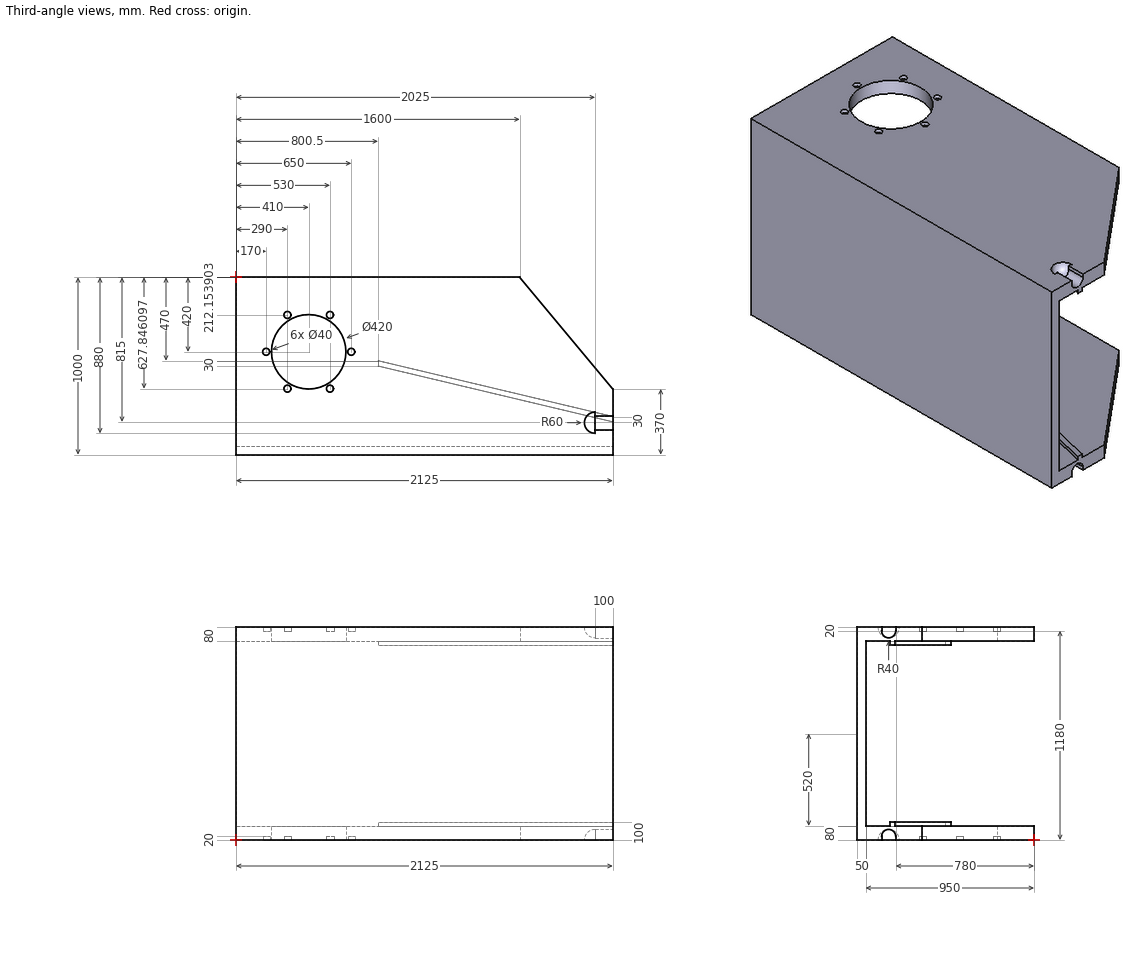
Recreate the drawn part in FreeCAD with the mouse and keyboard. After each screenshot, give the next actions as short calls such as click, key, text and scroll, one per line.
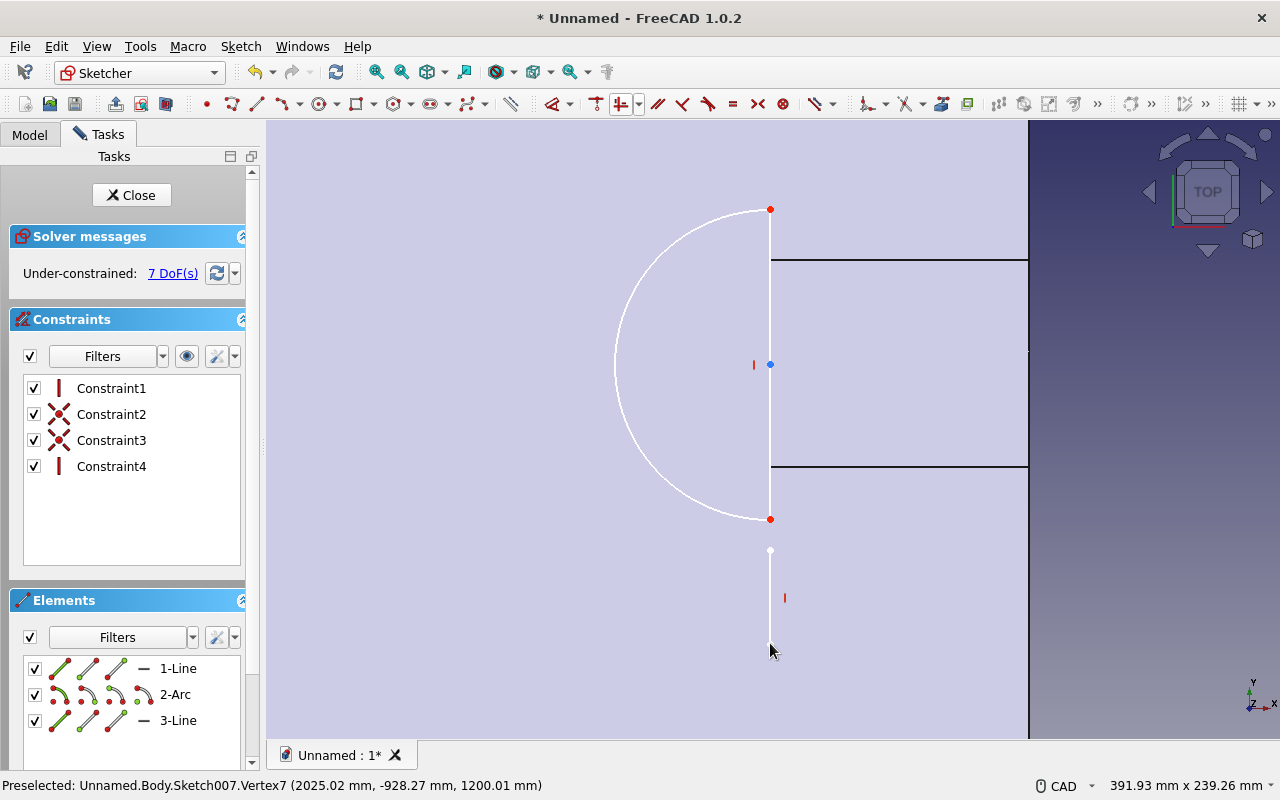
click(770, 579)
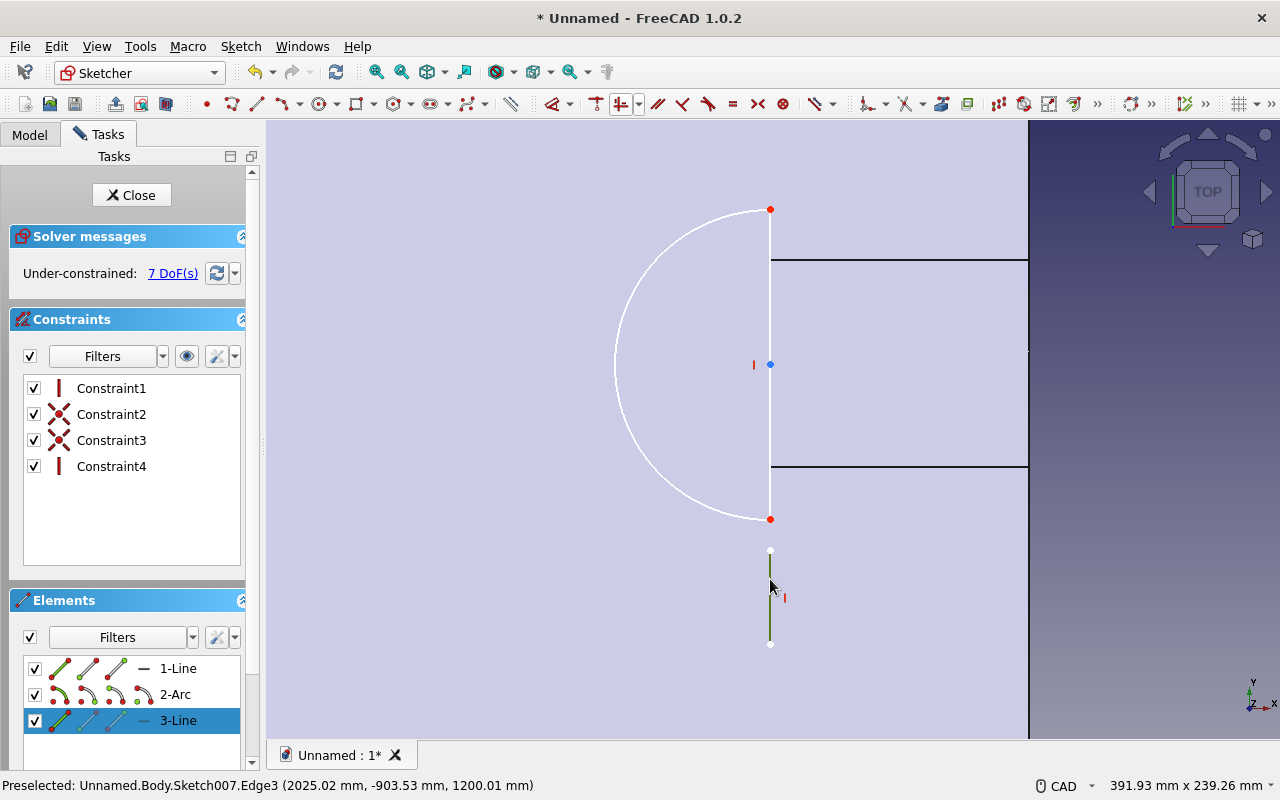
key(g)
key(n)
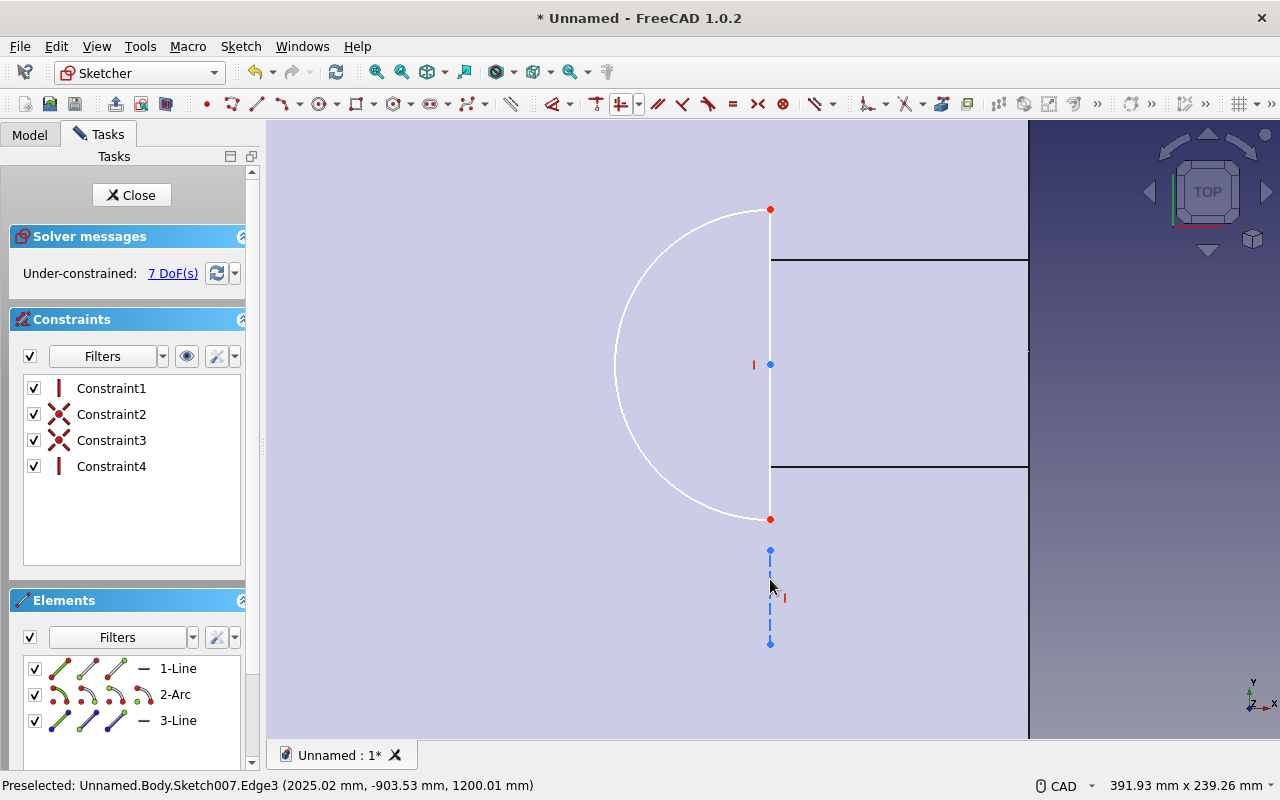
key(d)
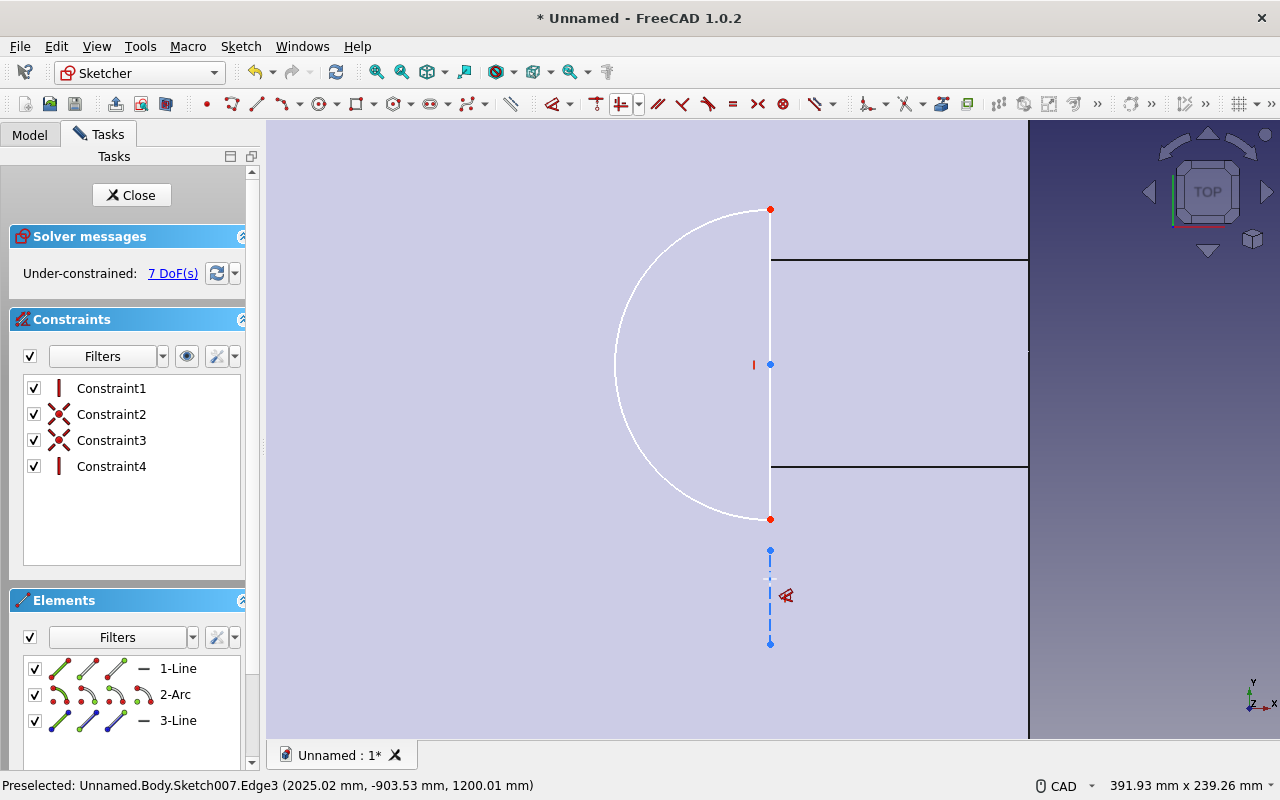
click(645, 274)
click(619, 255)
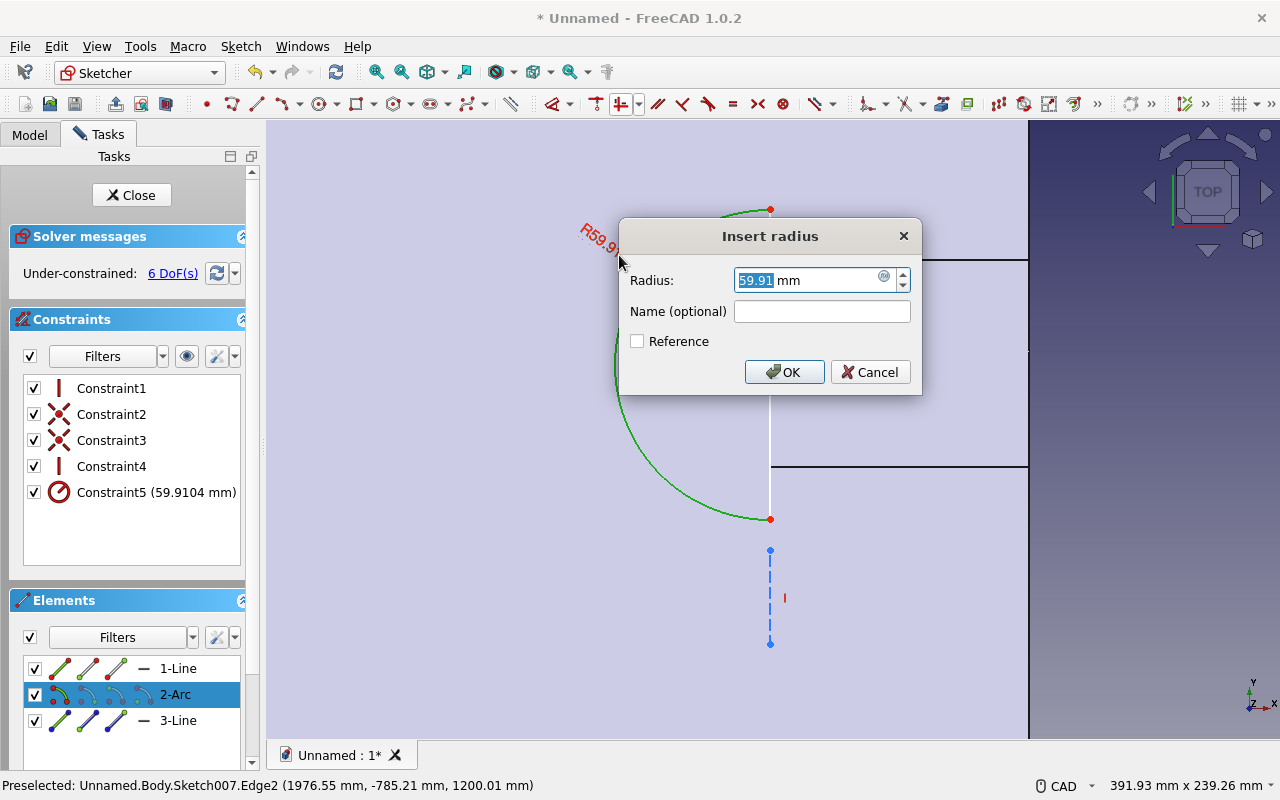
text(60)
key(Return)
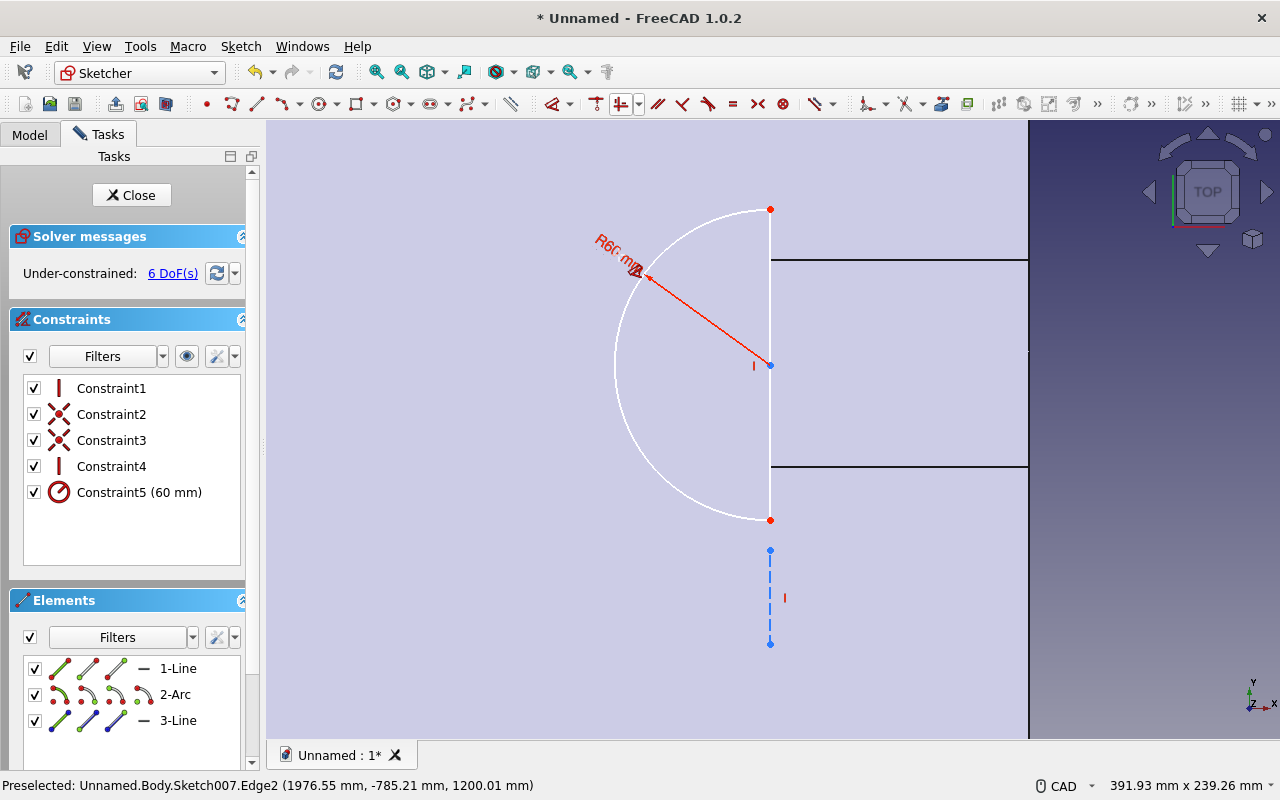
click(770, 520)
click(804, 334)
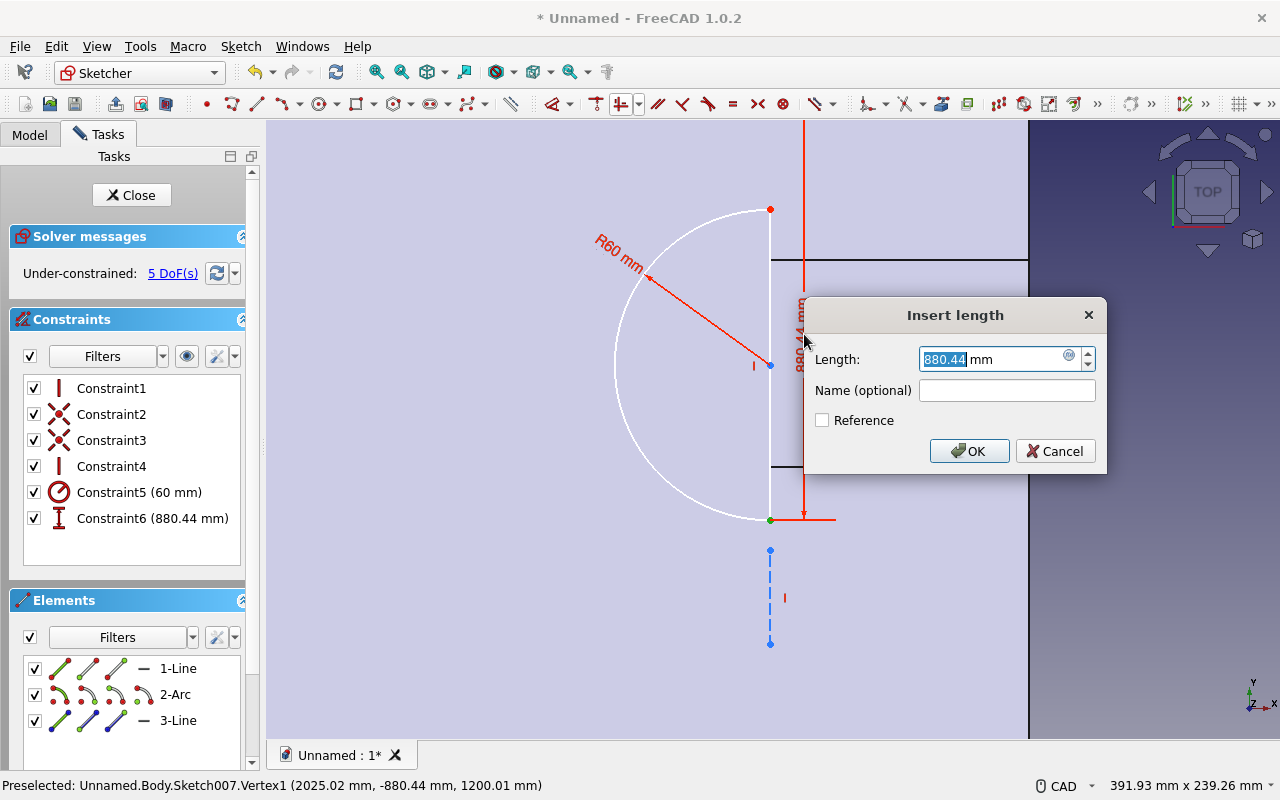
text(880)
key(Return)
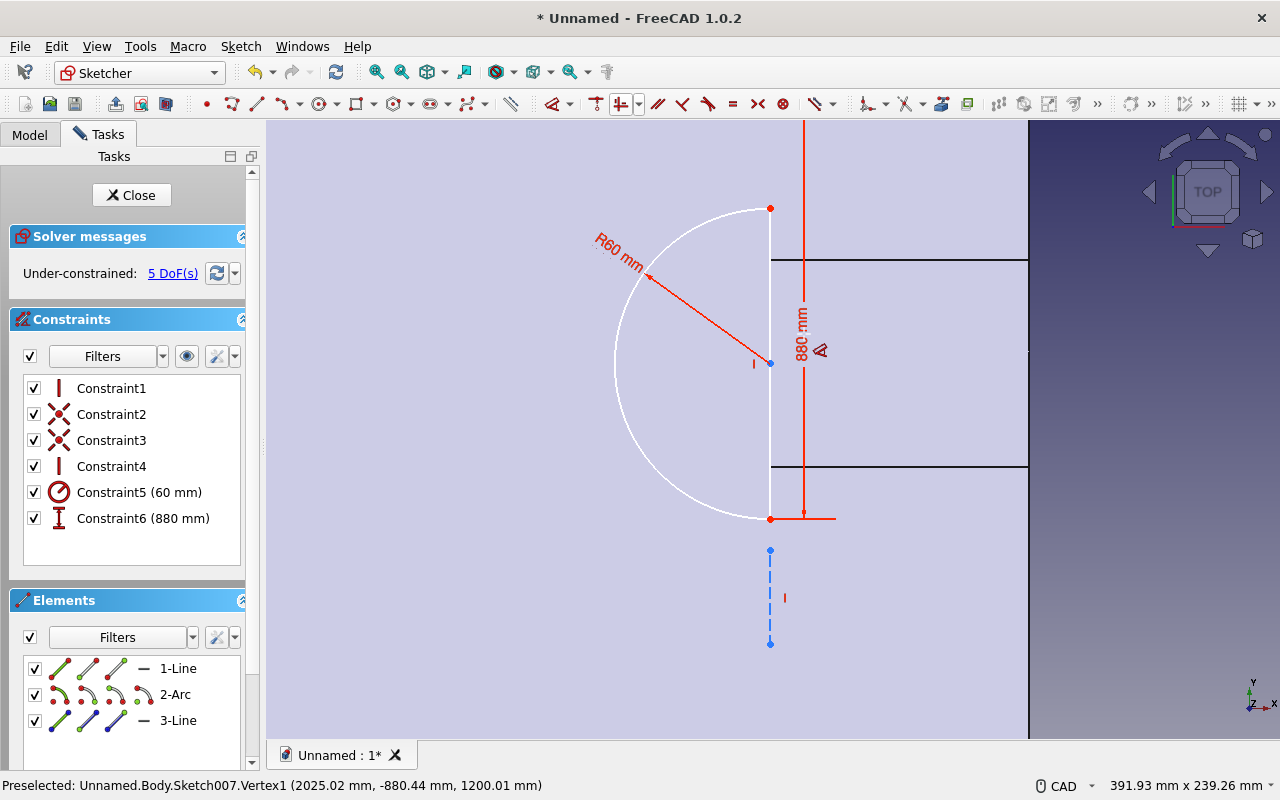
click(770, 519)
click(532, 553)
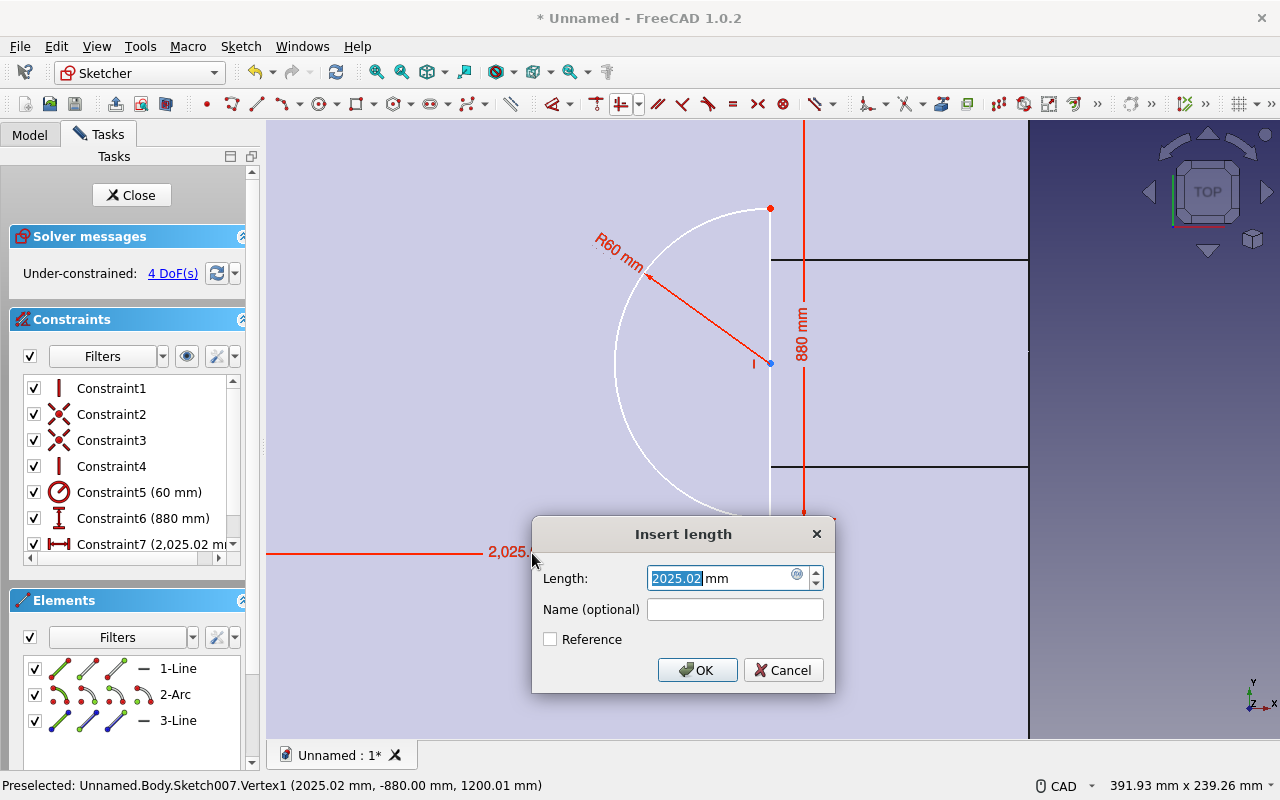
text(2025)
key(Return)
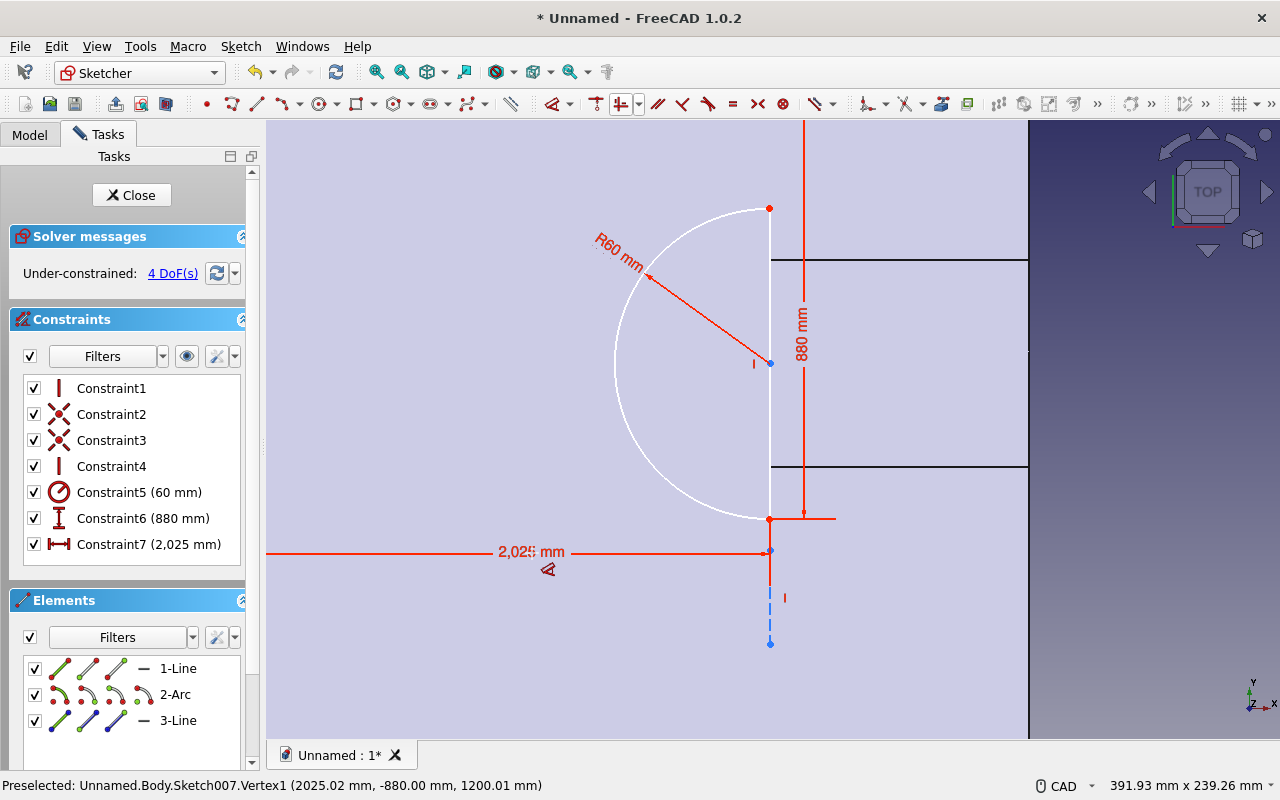
click(770, 551)
click(532, 585)